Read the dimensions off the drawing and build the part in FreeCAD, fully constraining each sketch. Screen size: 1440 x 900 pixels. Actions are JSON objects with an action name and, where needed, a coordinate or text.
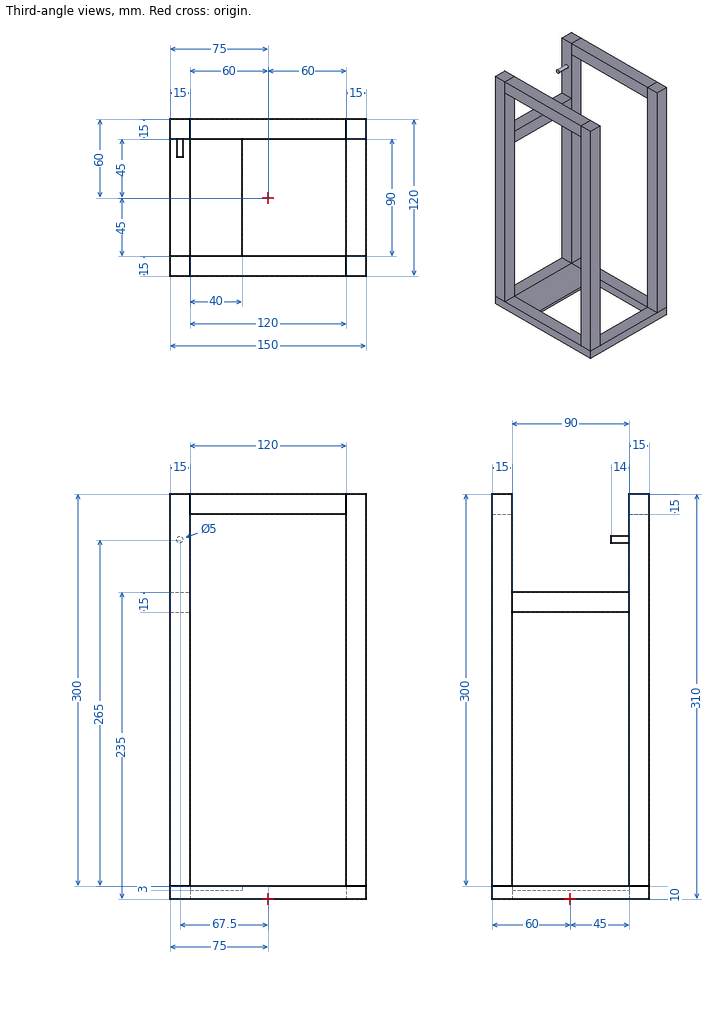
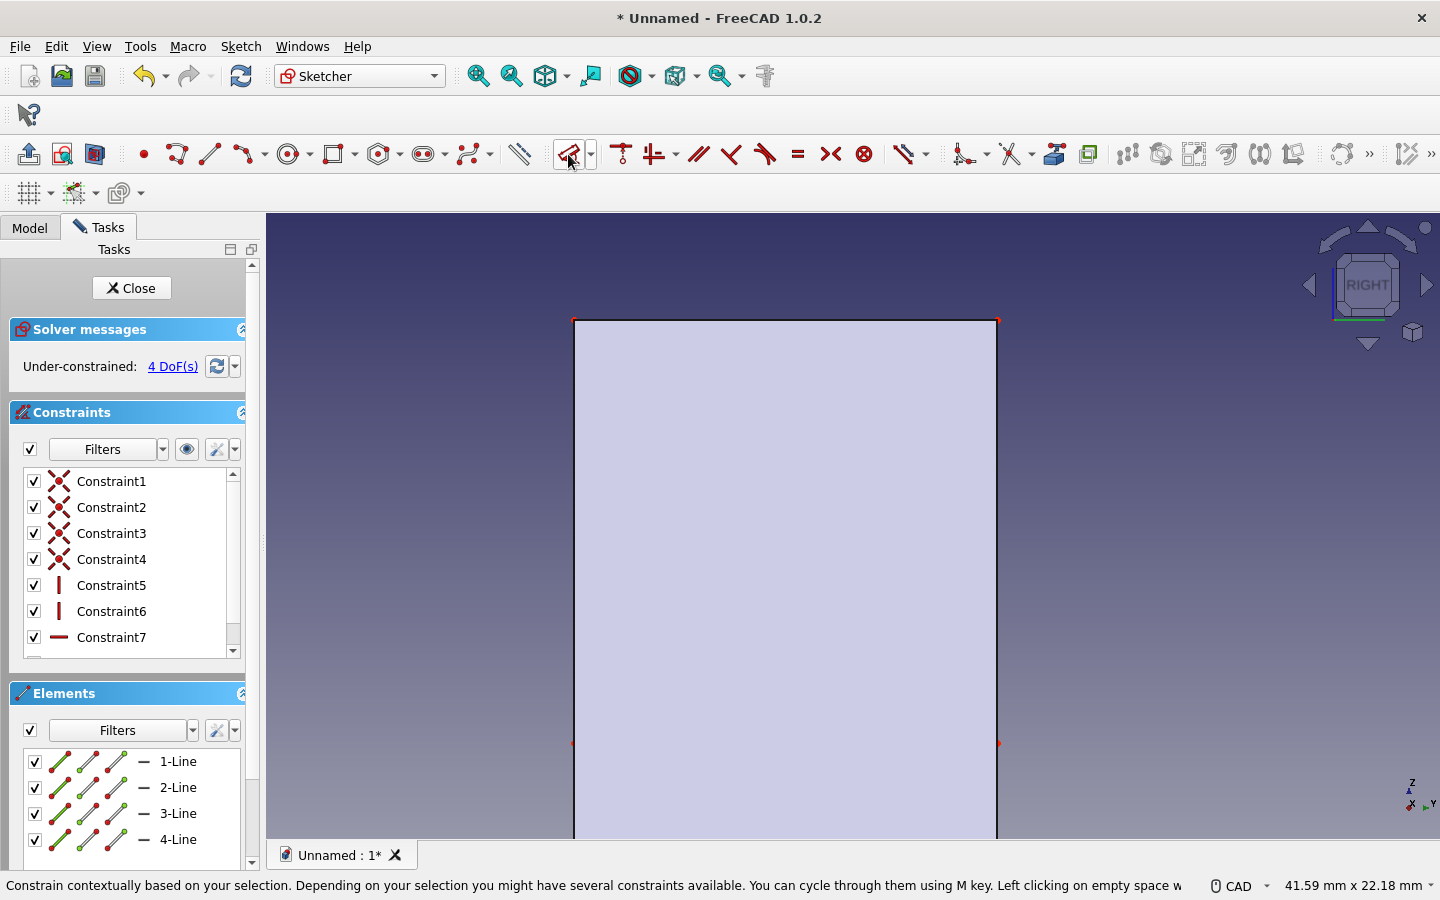
{"action": "left_click", "coordinate": [574, 448]}
{"action": "left_click", "coordinate": [540, 532]}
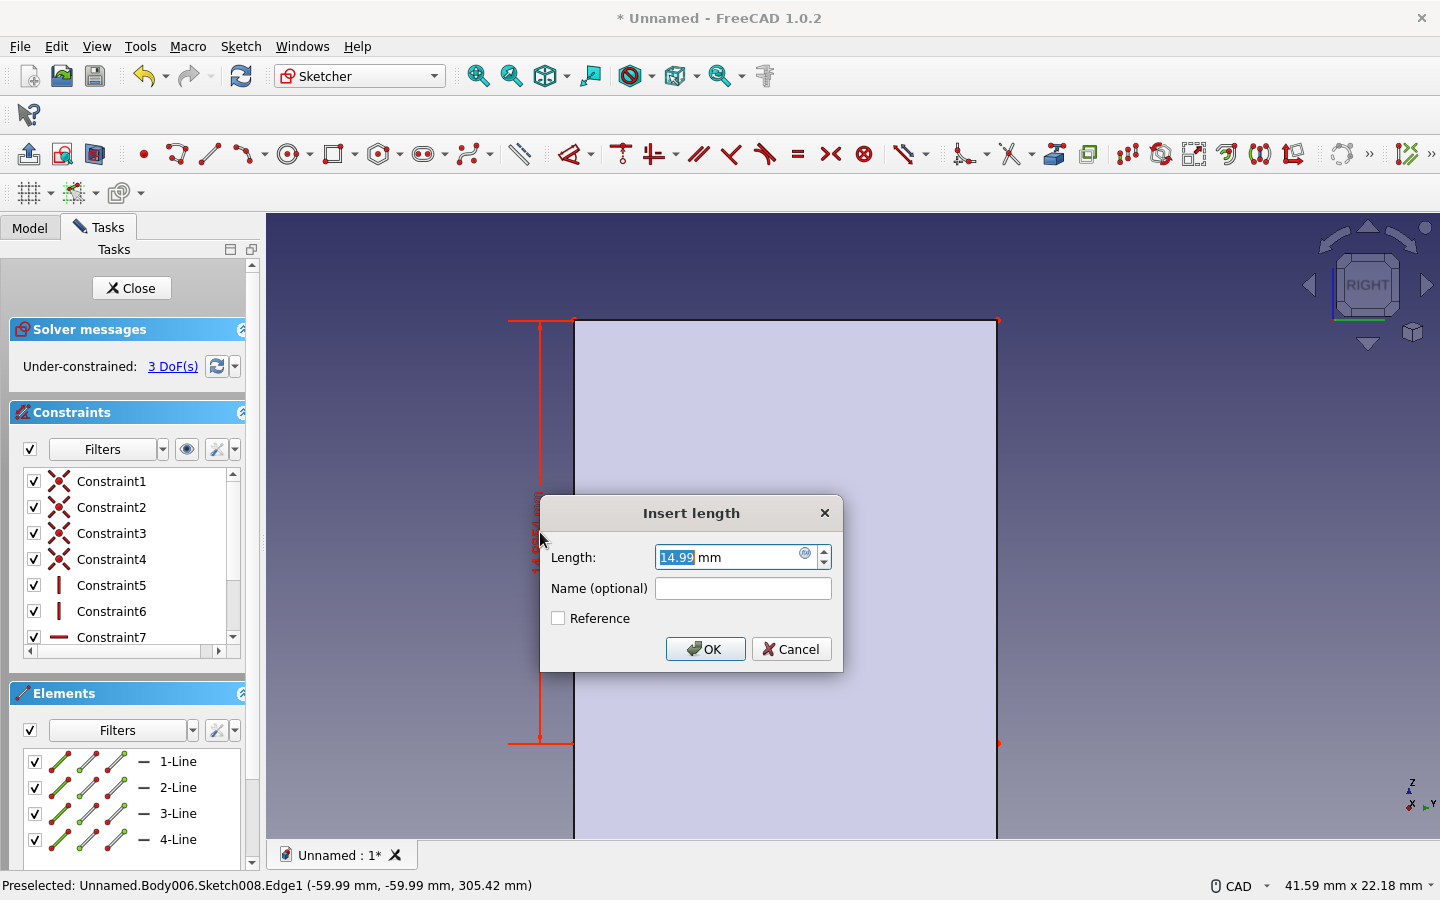
{"action": "type", "text": "15"}
{"action": "key", "text": "Return"}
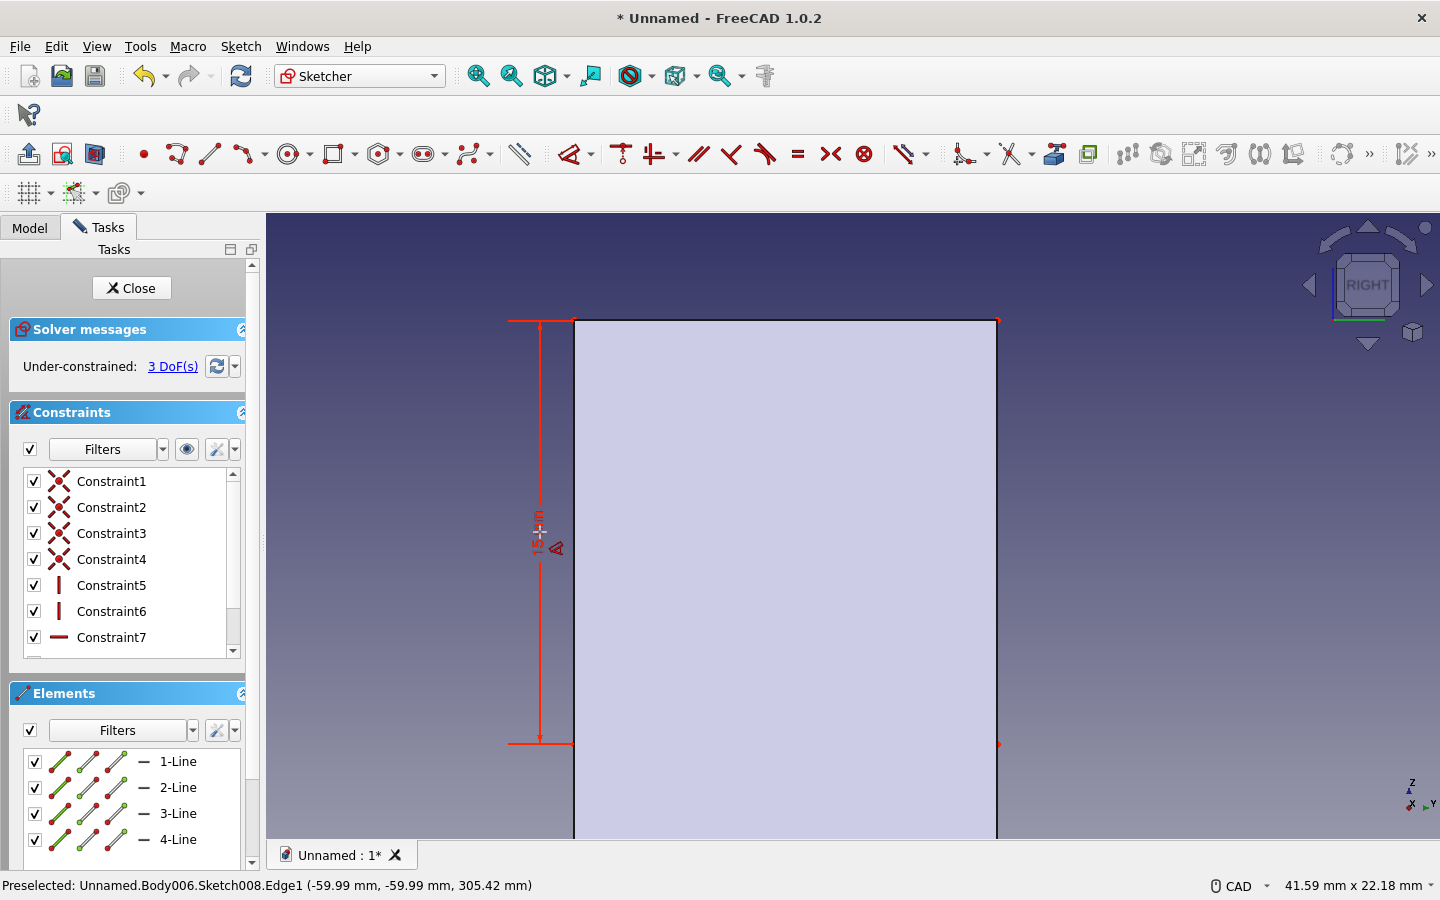
{"action": "left_click", "coordinate": [701, 744]}
{"action": "left_click", "coordinate": [786, 778]}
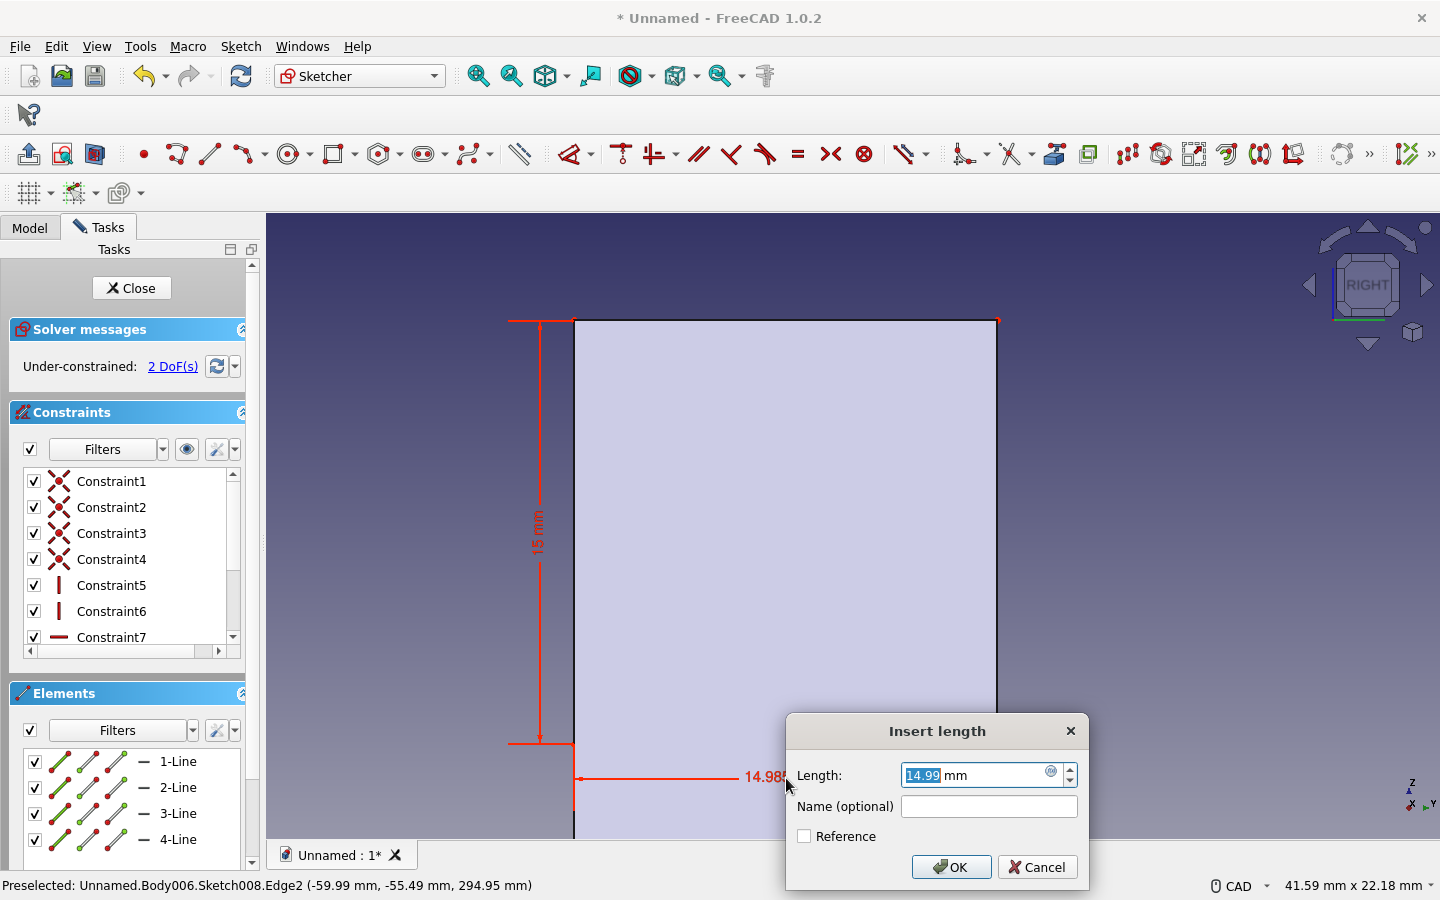
{"action": "type", "text": "15"}
{"action": "key", "text": "Return"}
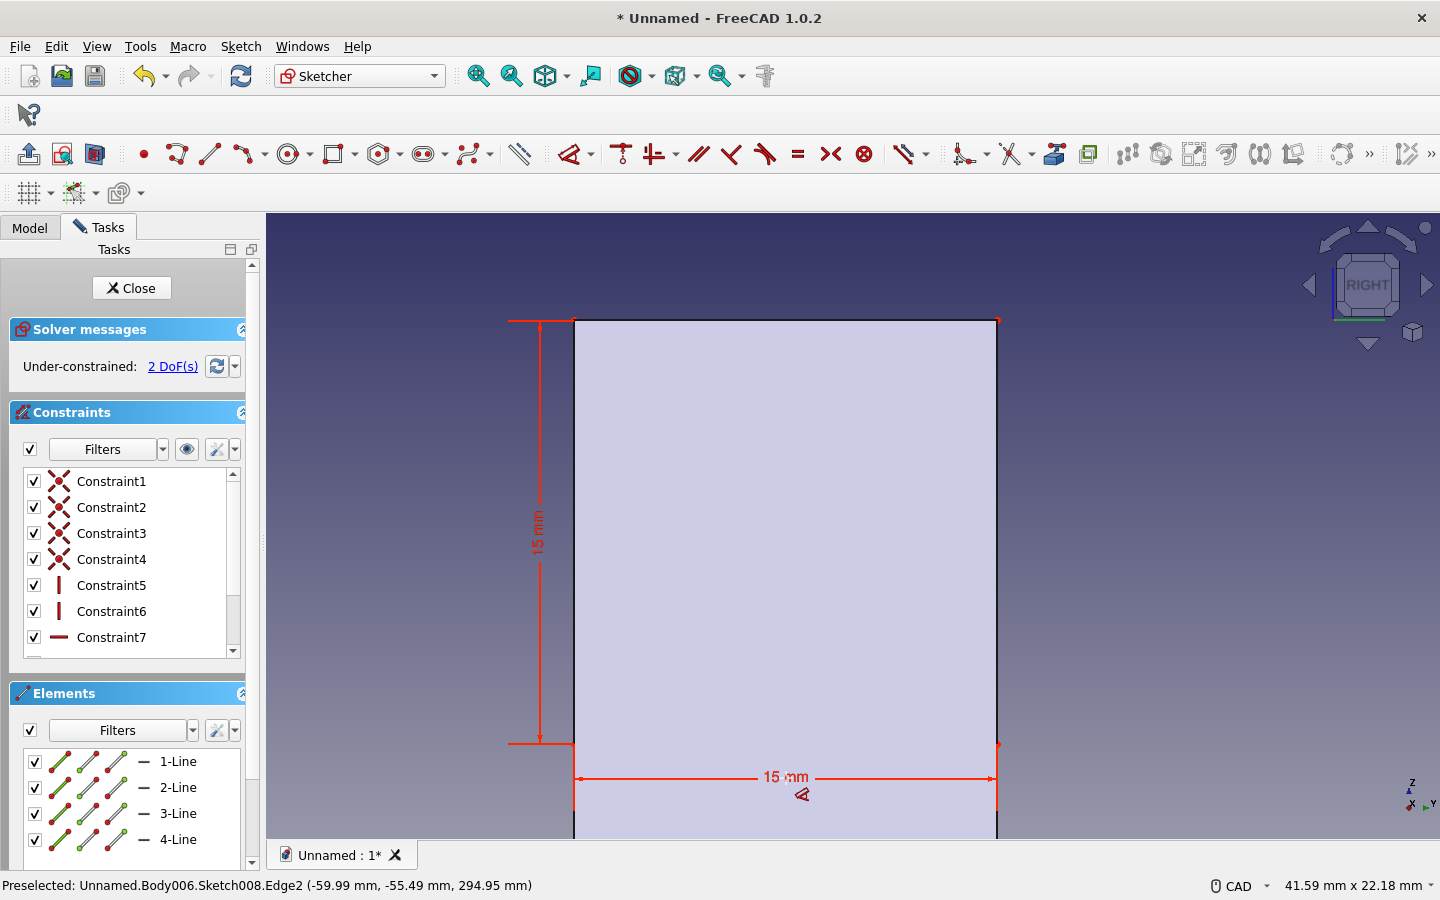
{"action": "left_click", "coordinate": [574, 321]}
{"action": "left_click", "coordinate": [925, 287]}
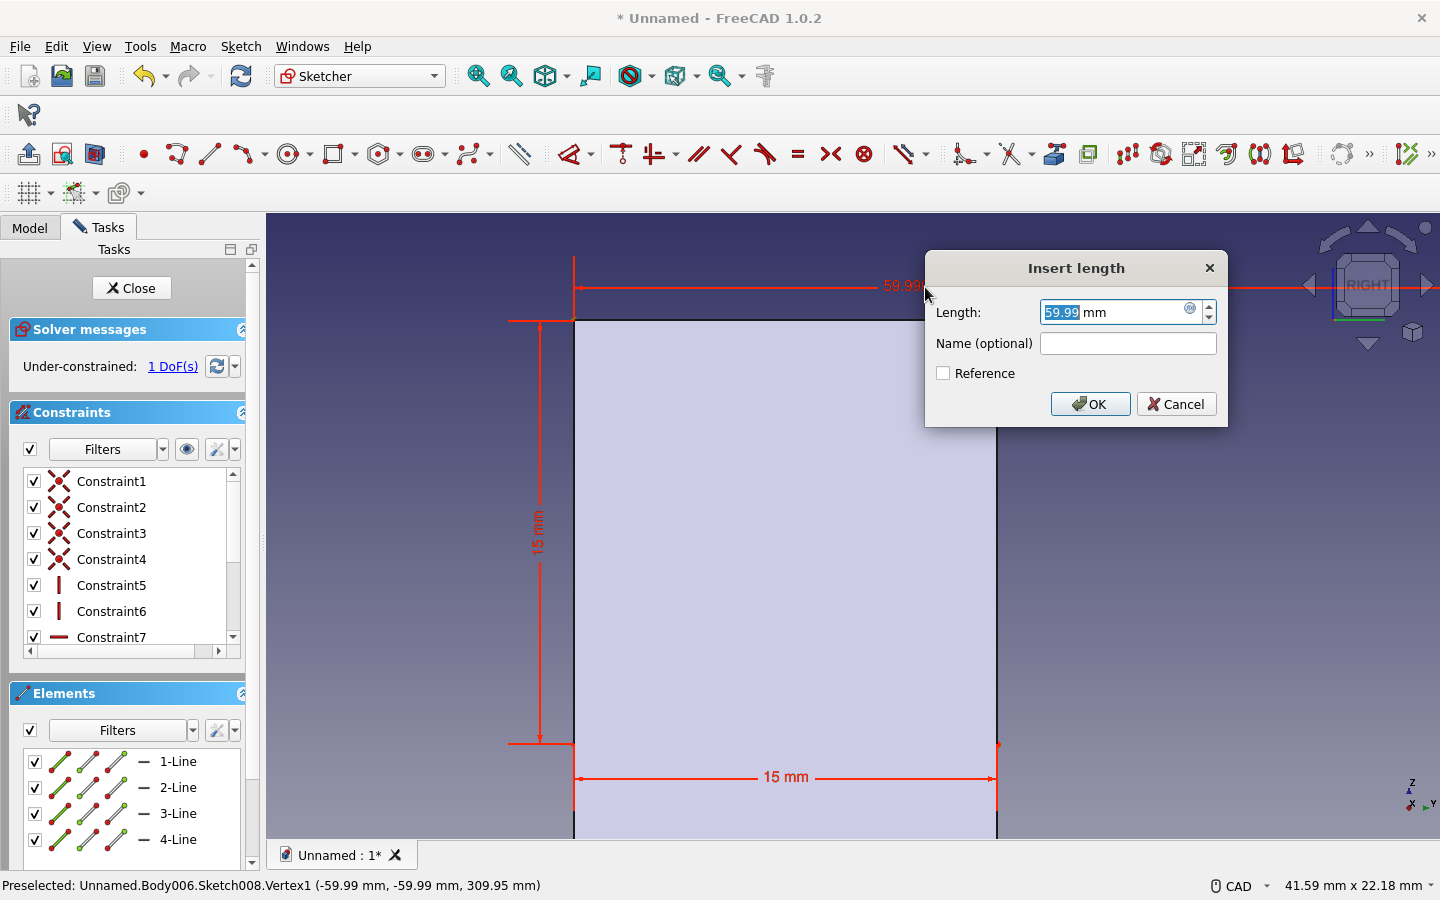
{"action": "type", "text": "60"}
{"action": "key", "text": "Return"}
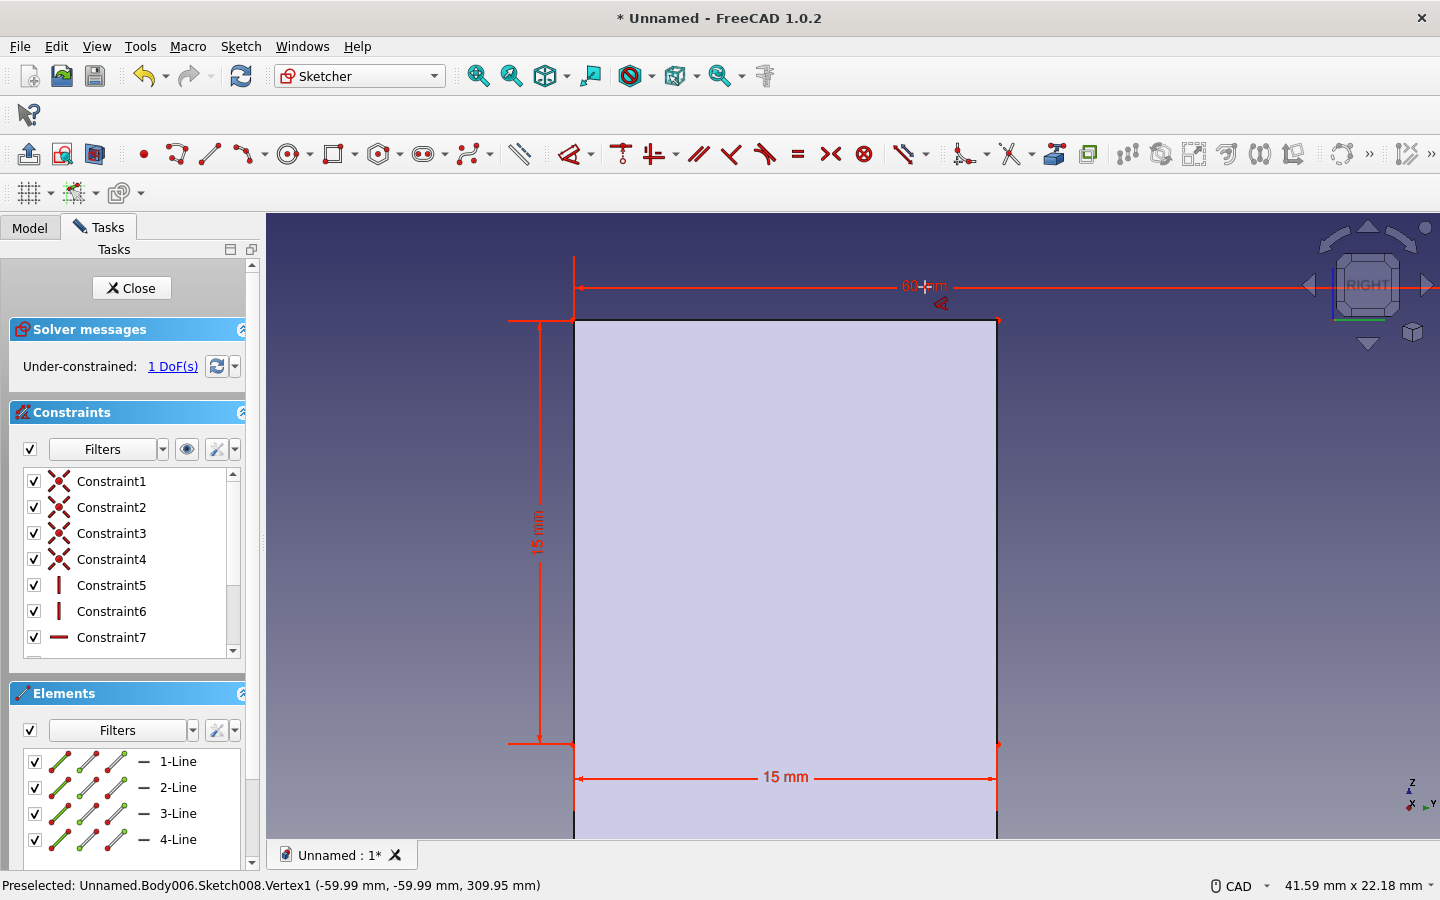
{"action": "left_click", "coordinate": [574, 321]}
{"action": "left_click", "coordinate": [540, 566]}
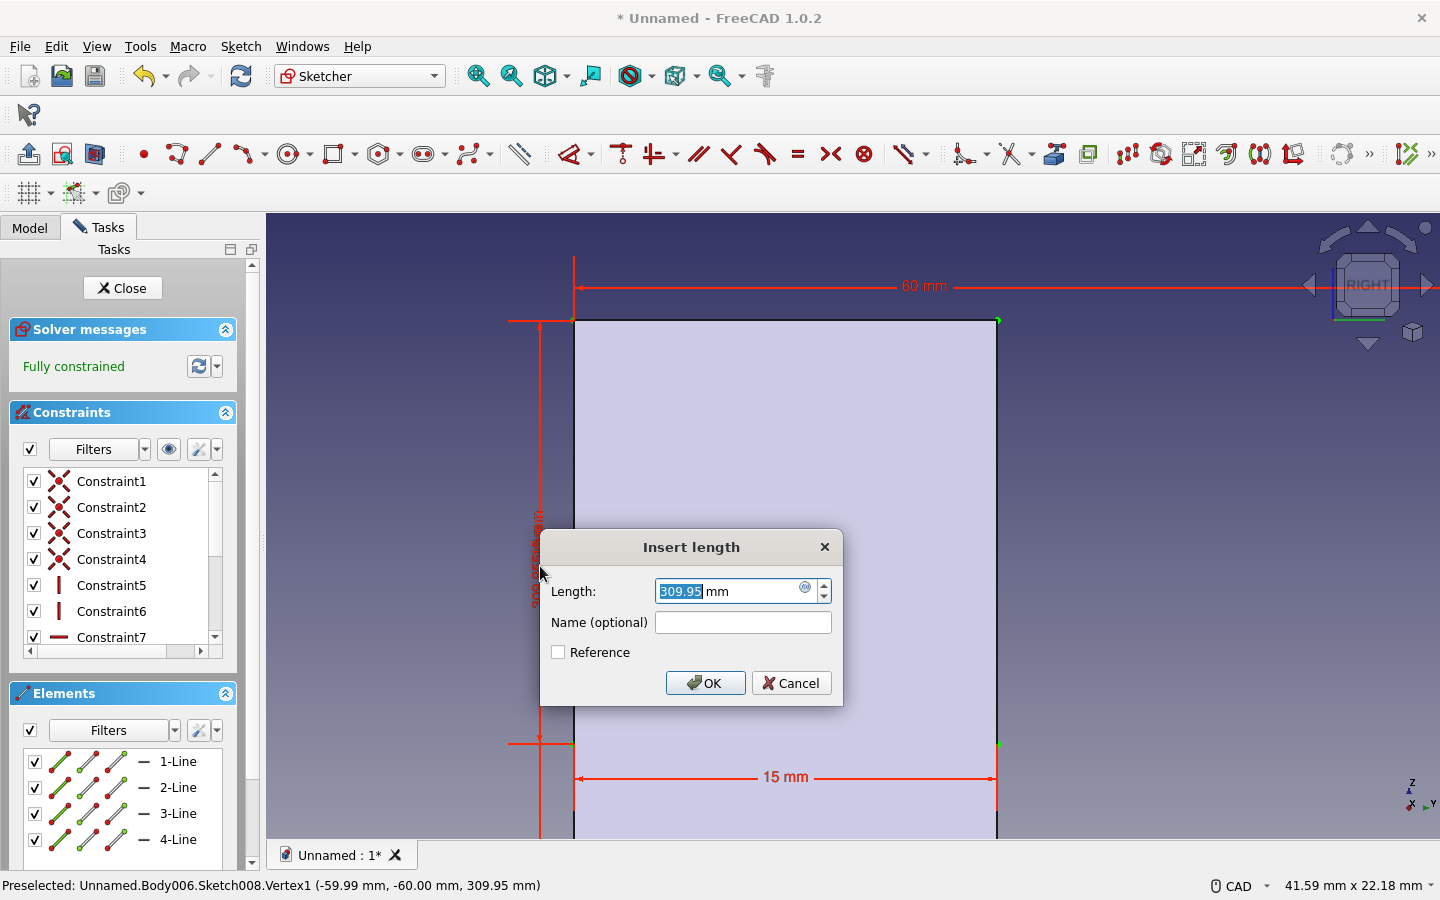
{"action": "type", "text": "310"}
{"action": "key", "text": "Return"}
{"action": "key", "text": "Escape"}